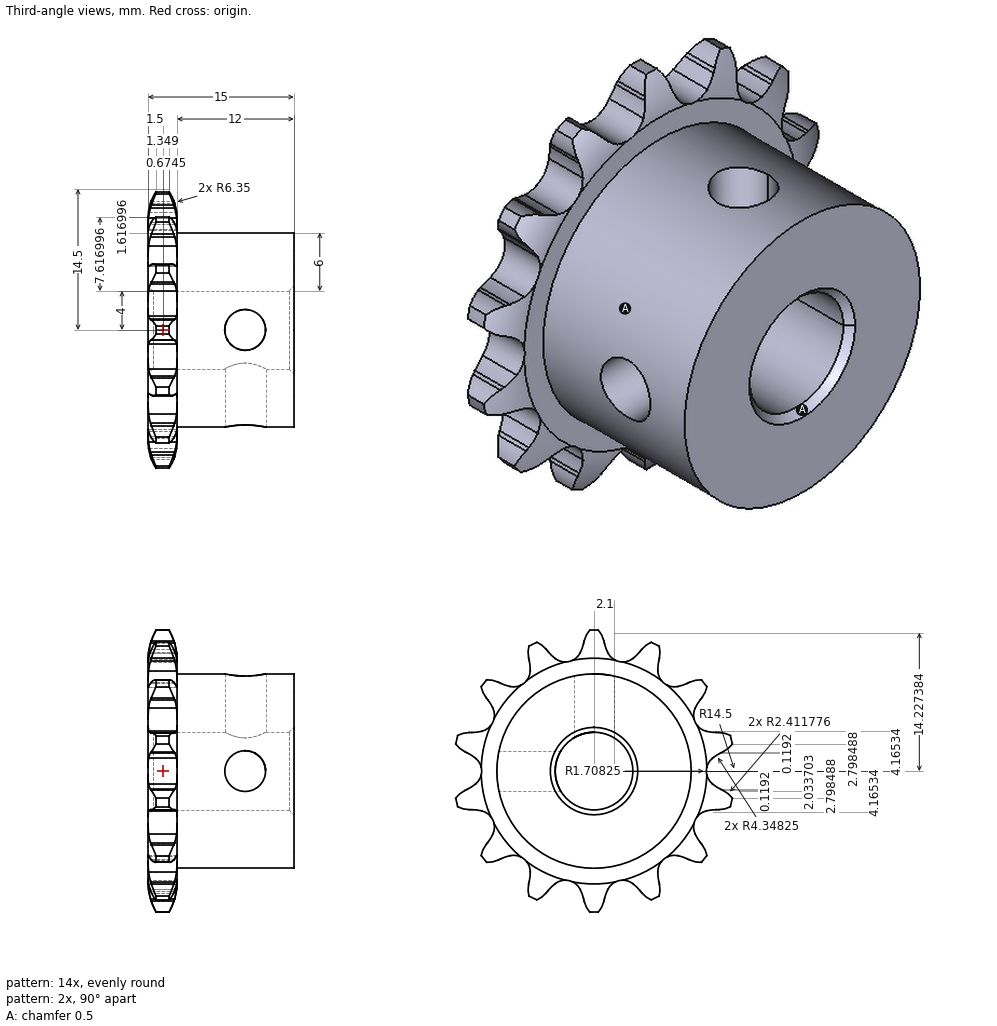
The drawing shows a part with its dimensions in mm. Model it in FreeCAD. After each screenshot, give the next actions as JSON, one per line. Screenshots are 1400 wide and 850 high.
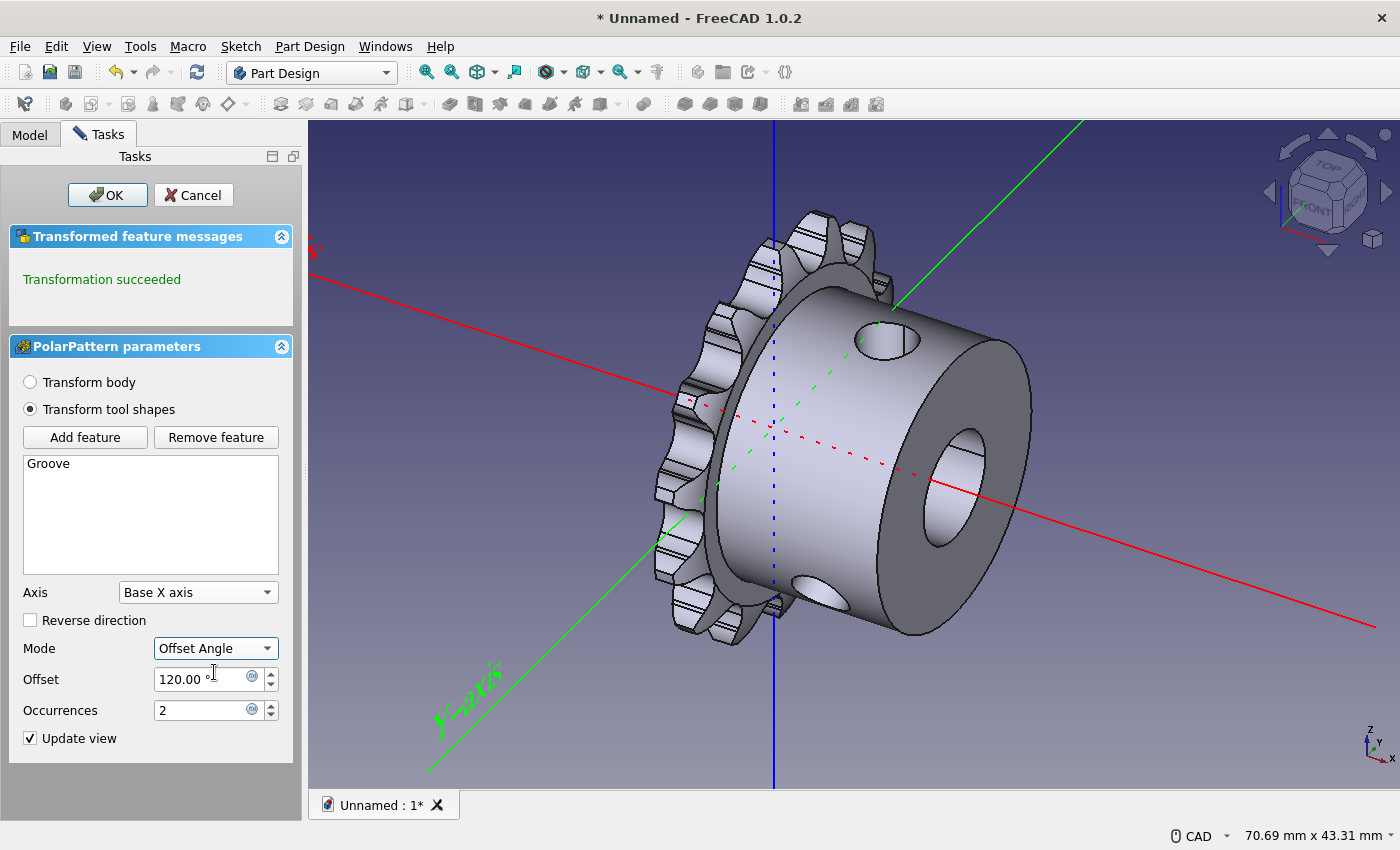
{"action": "triple_click", "coordinate": [210, 680]}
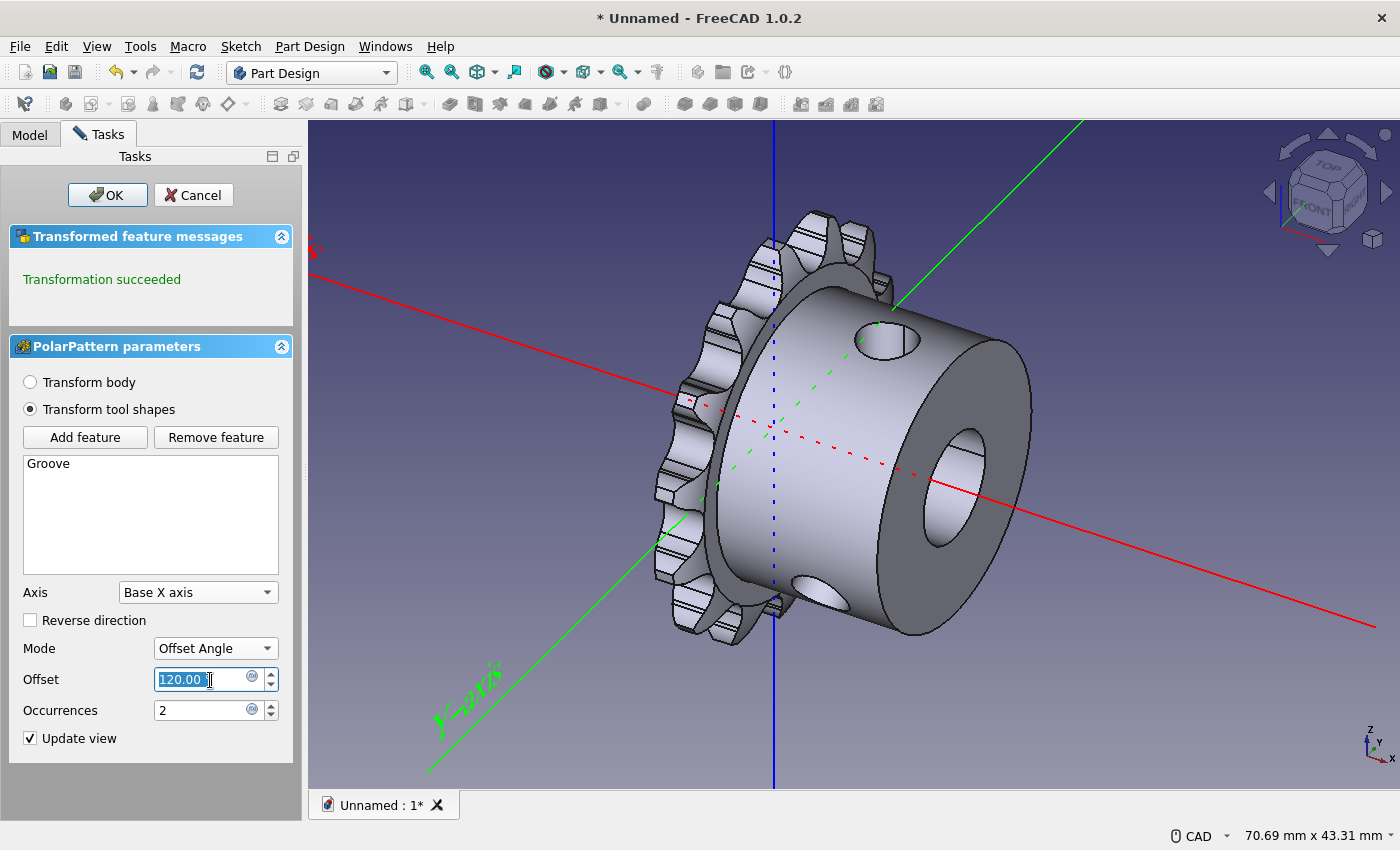
{"action": "type", "text": "90"}
{"action": "key", "text": "Tab"}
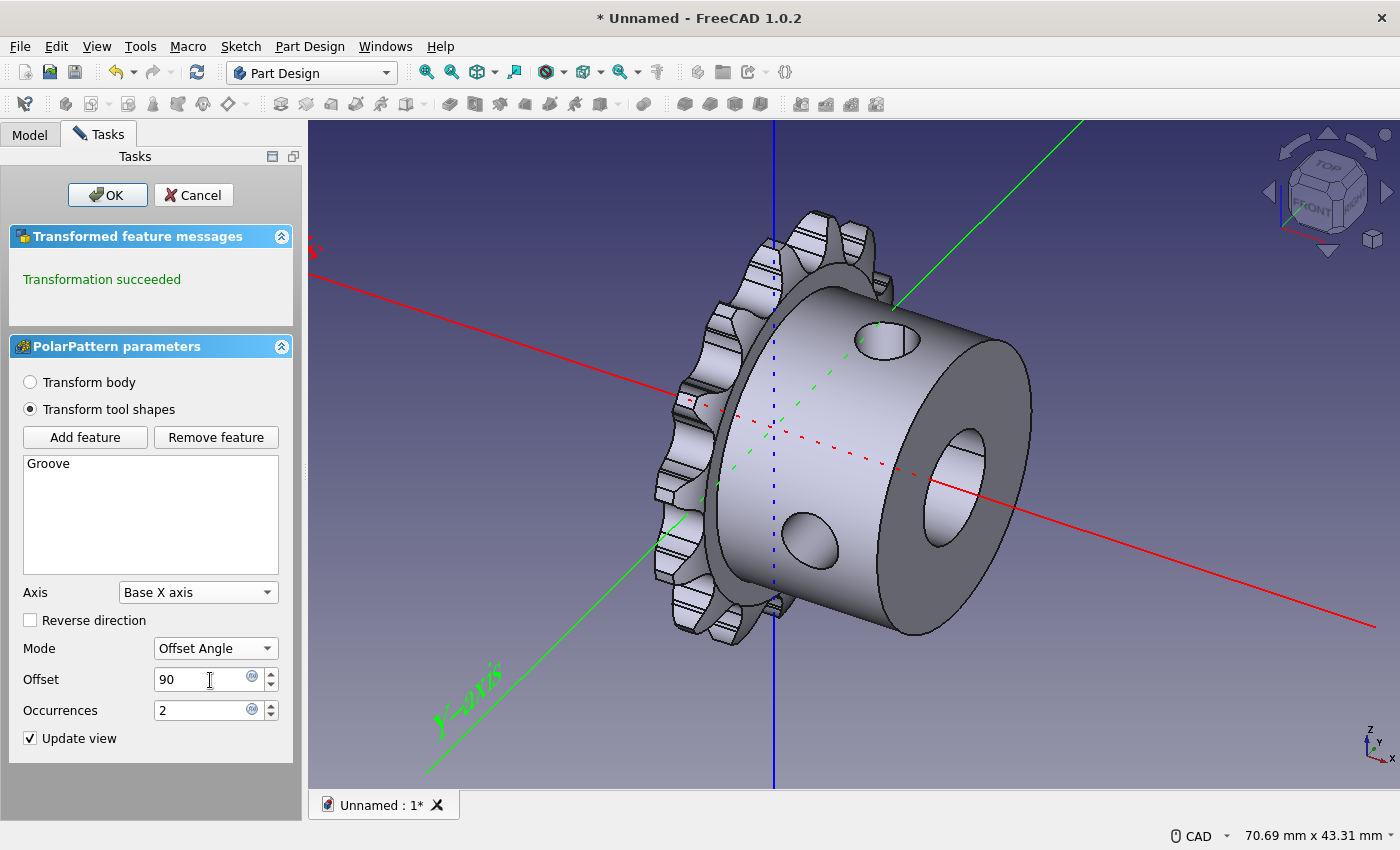
{"action": "triple_click", "coordinate": [210, 710]}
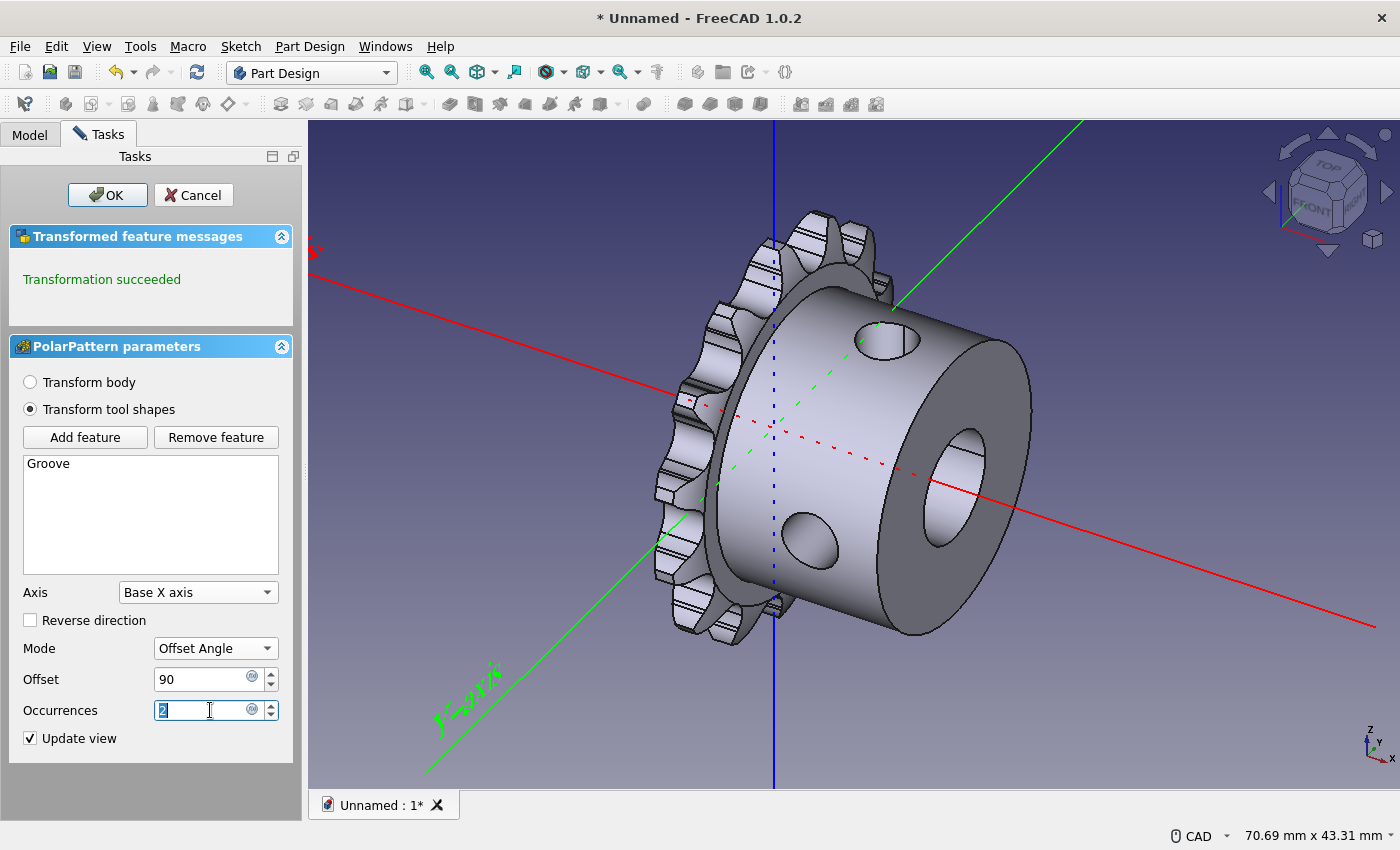
{"action": "type", "text": "2"}
{"action": "key", "text": "Tab"}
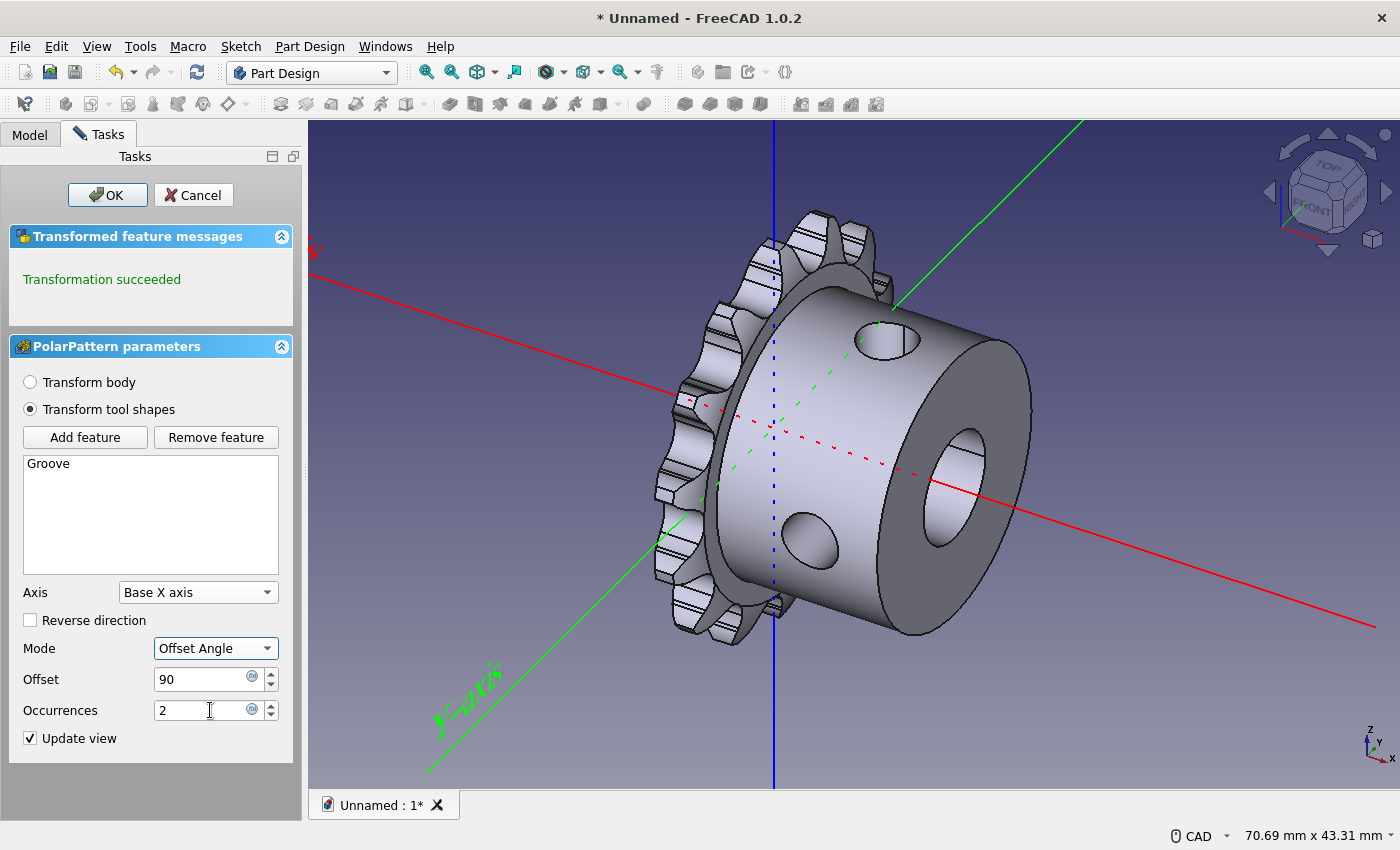
{"action": "left_click", "coordinate": [108, 195]}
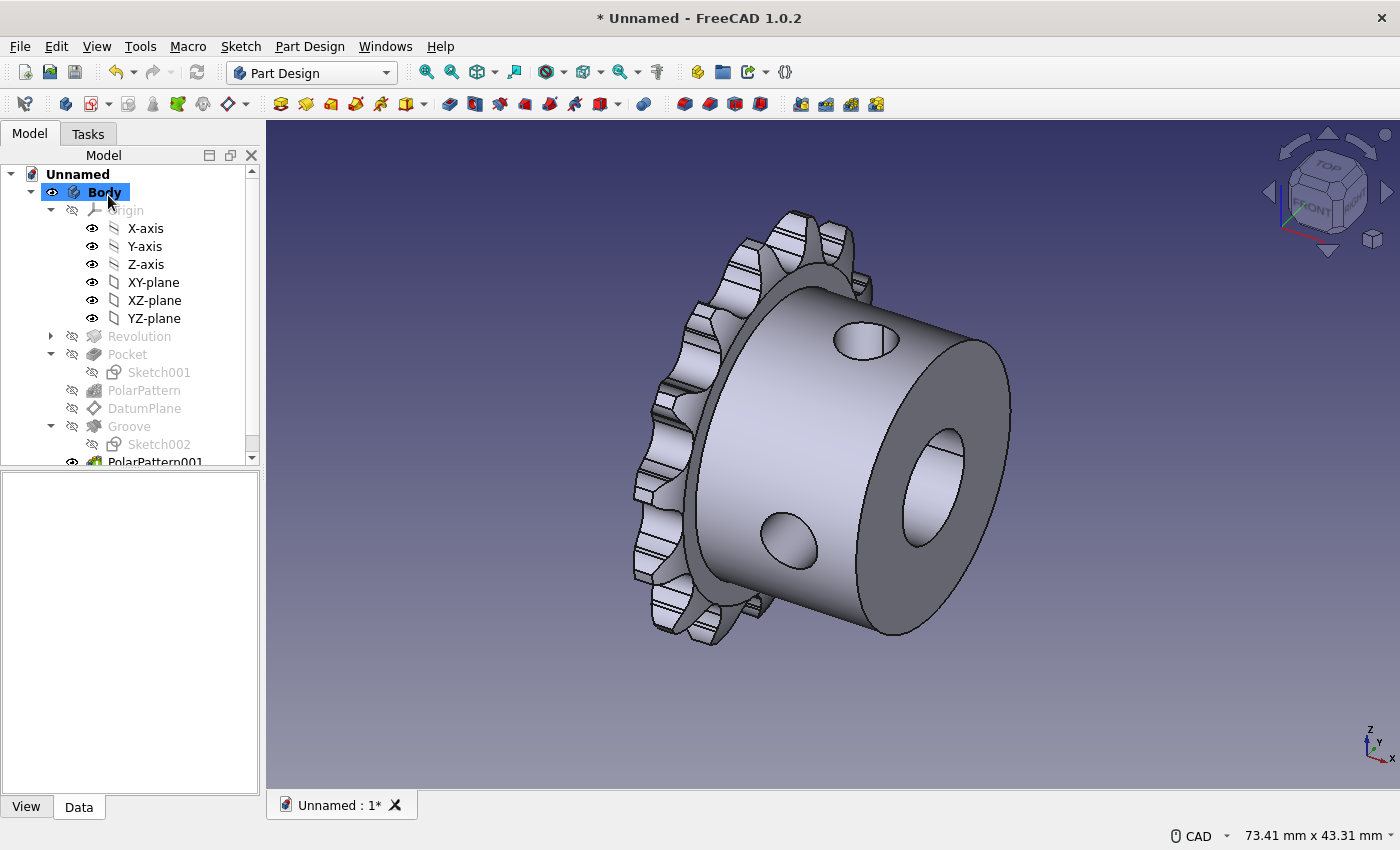
{"action": "left_click", "coordinate": [924, 544]}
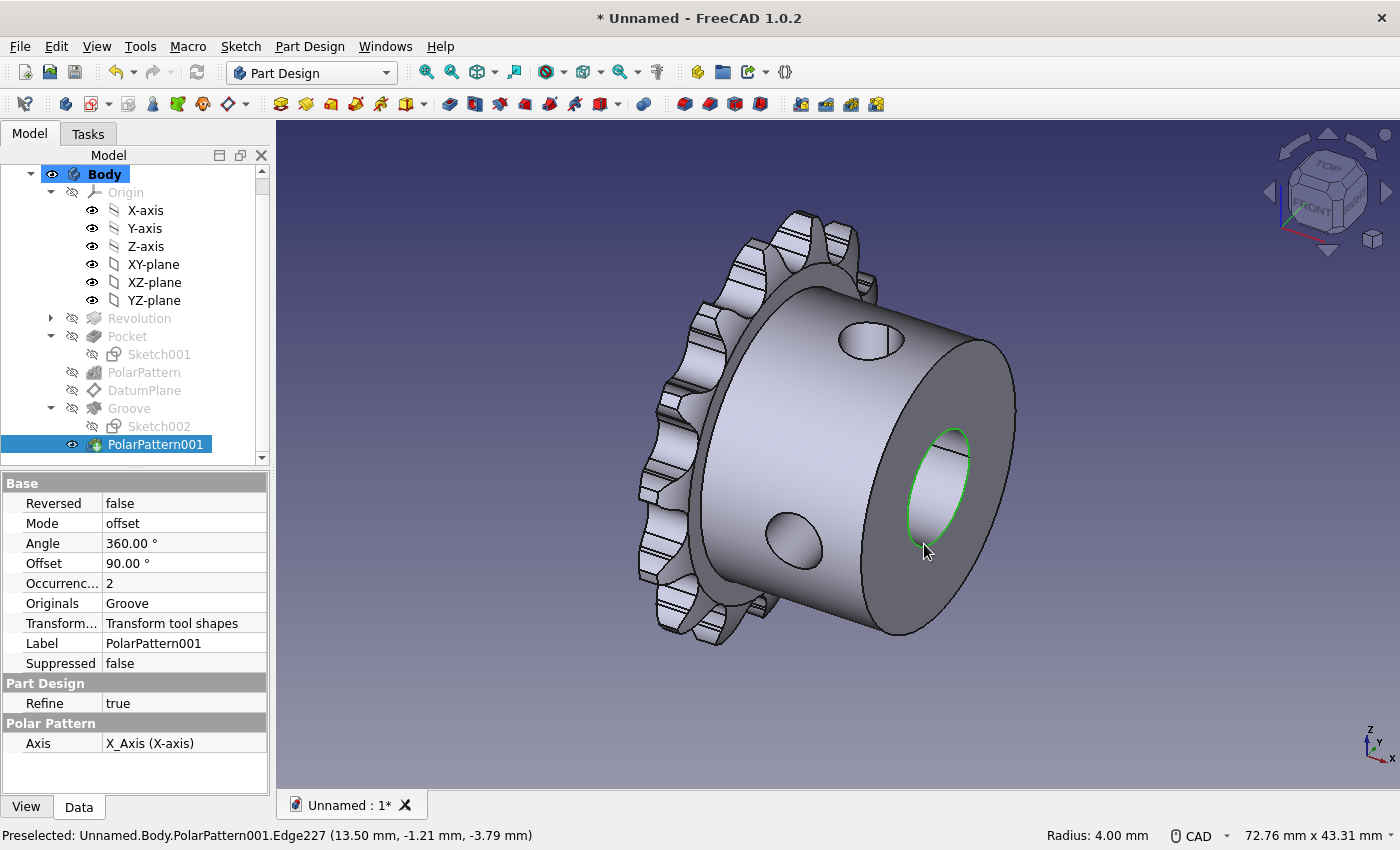
{"action": "key", "text": "0"}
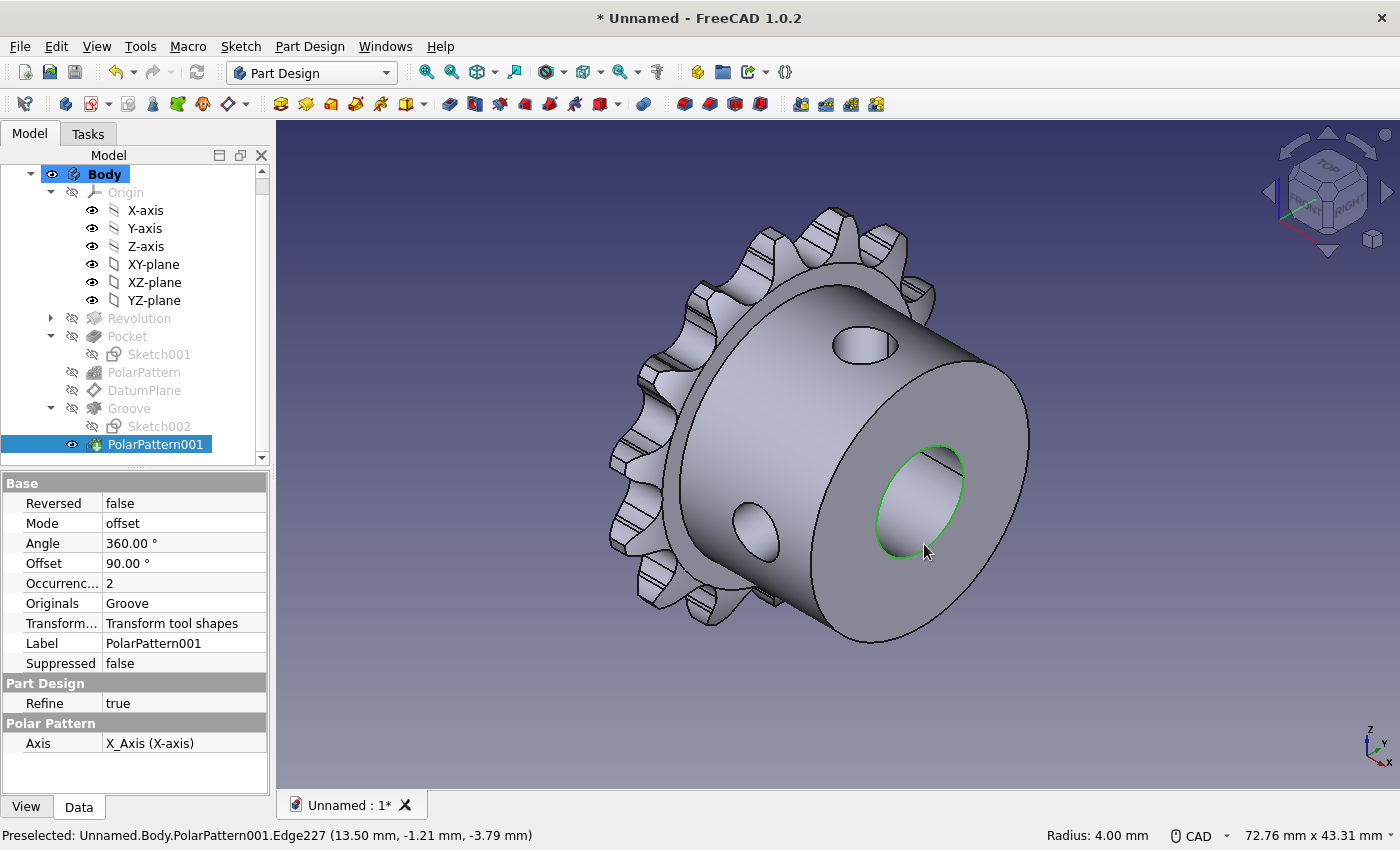
{"action": "key", "text": "2"}